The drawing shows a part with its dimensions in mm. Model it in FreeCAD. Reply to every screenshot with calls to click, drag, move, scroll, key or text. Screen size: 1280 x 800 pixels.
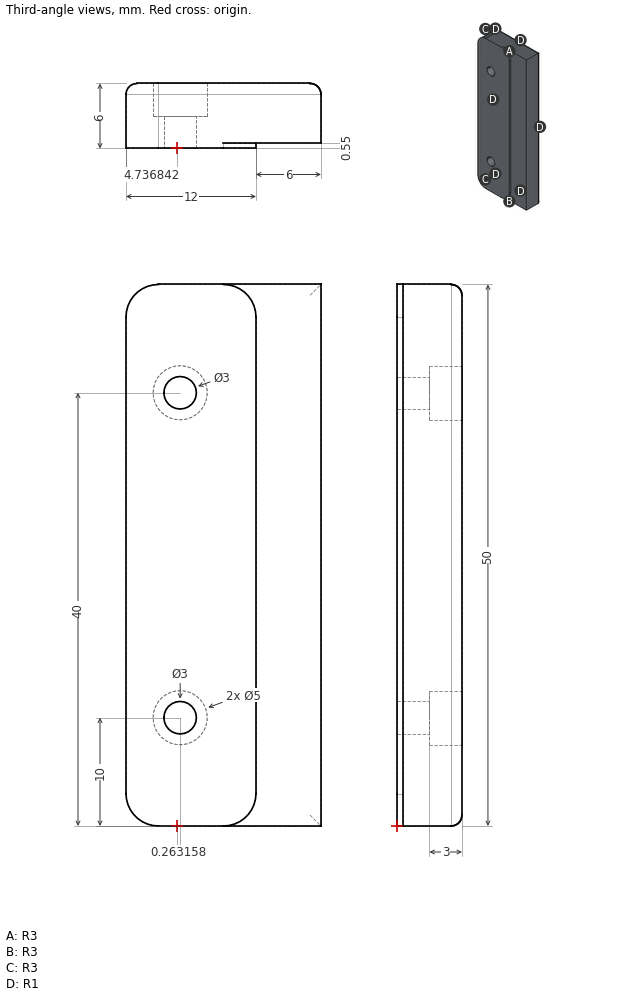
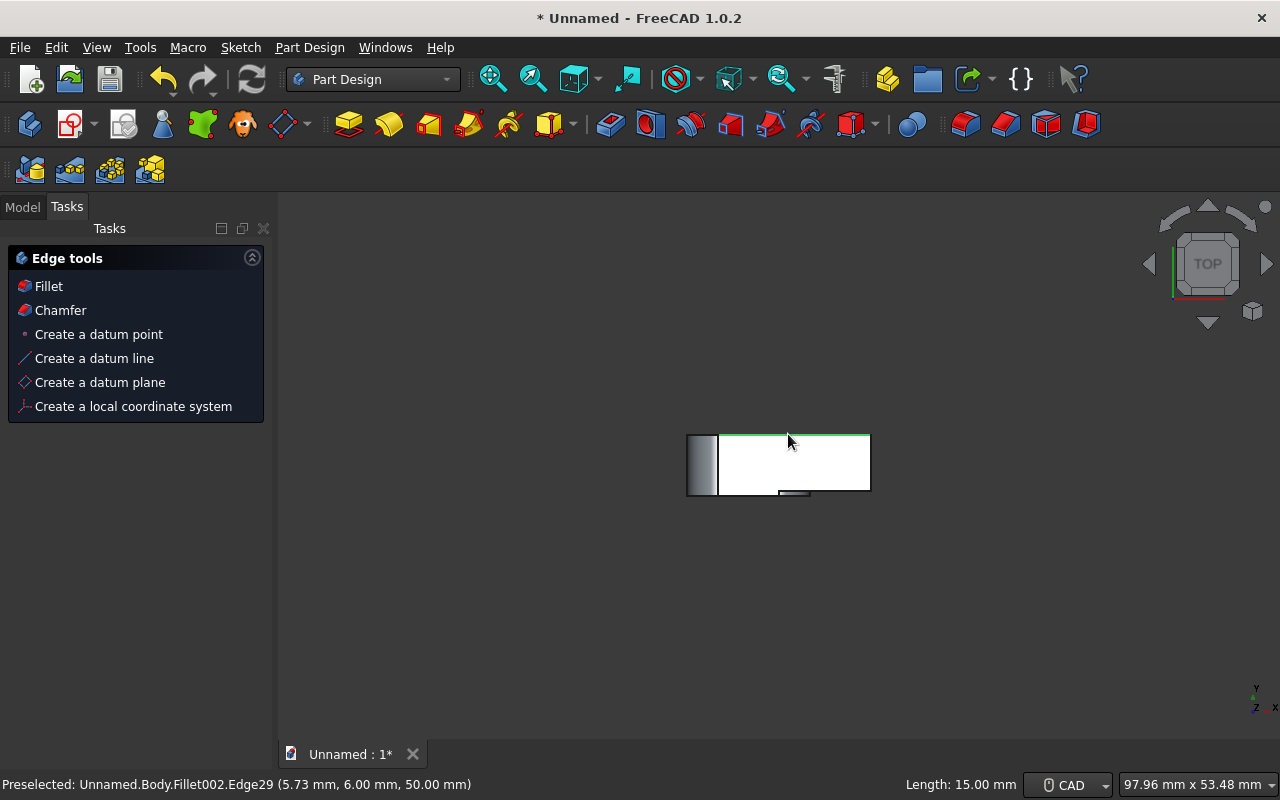
click(696, 434, ctrl)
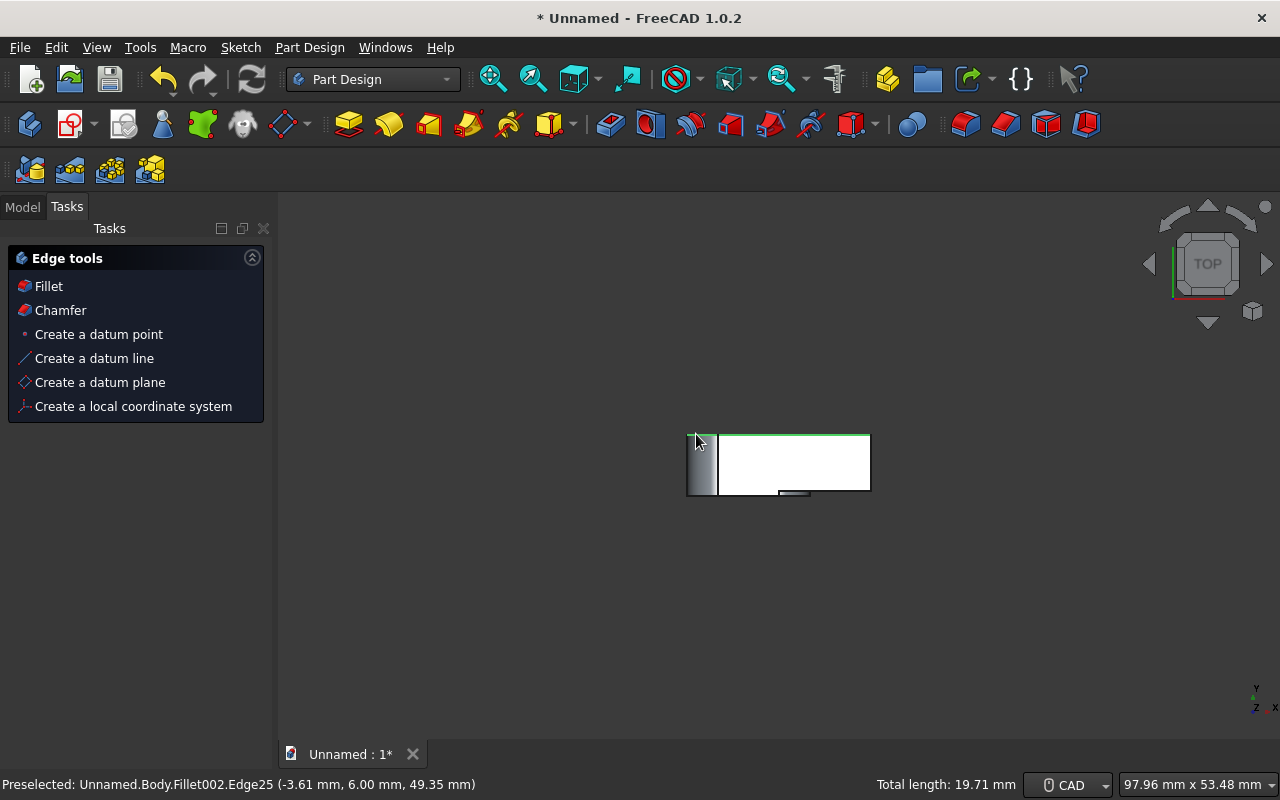
key(0)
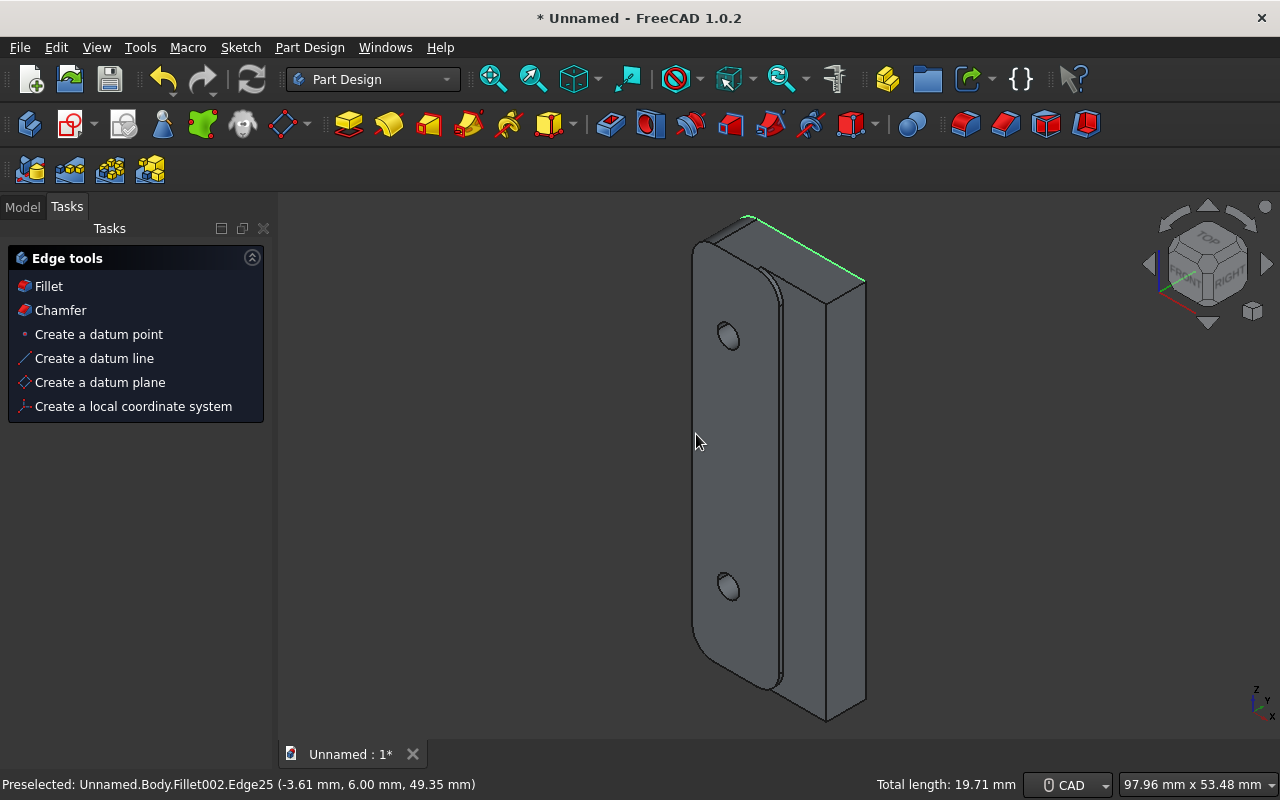
key(1)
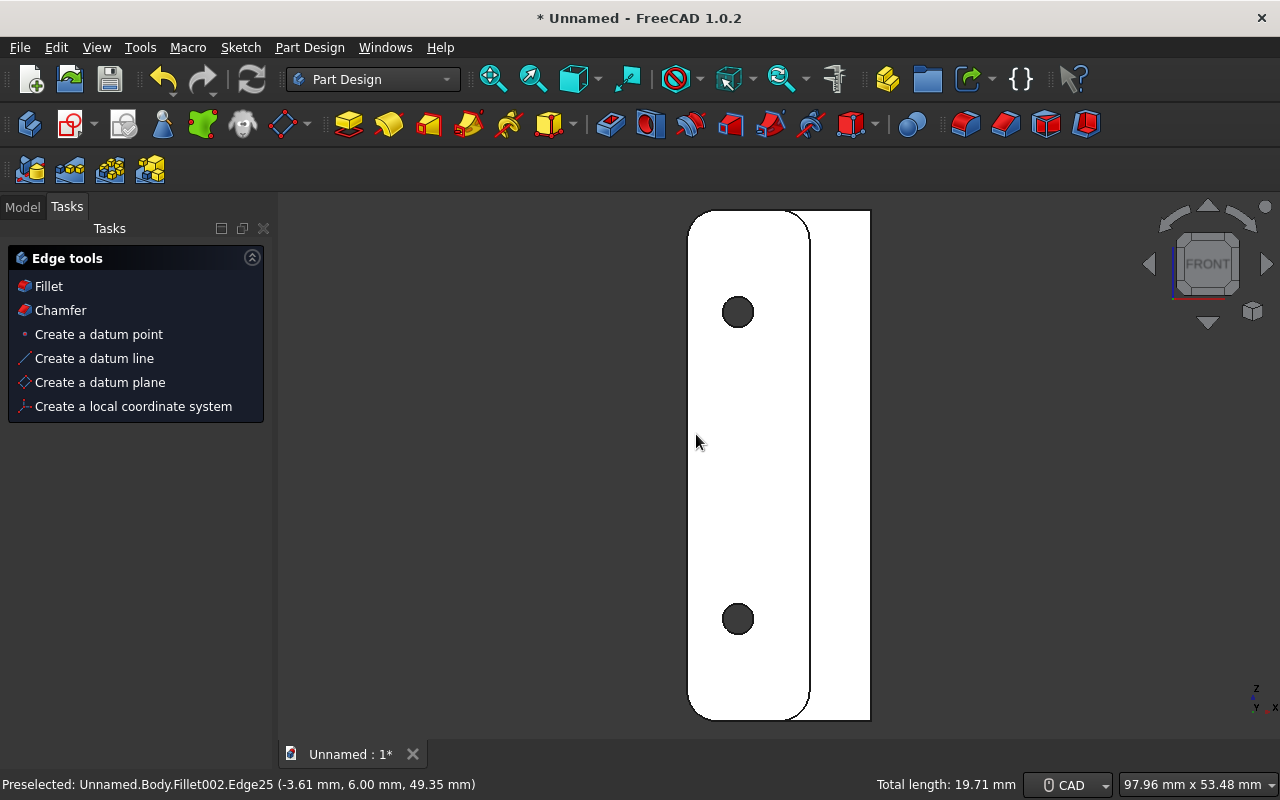
key(3)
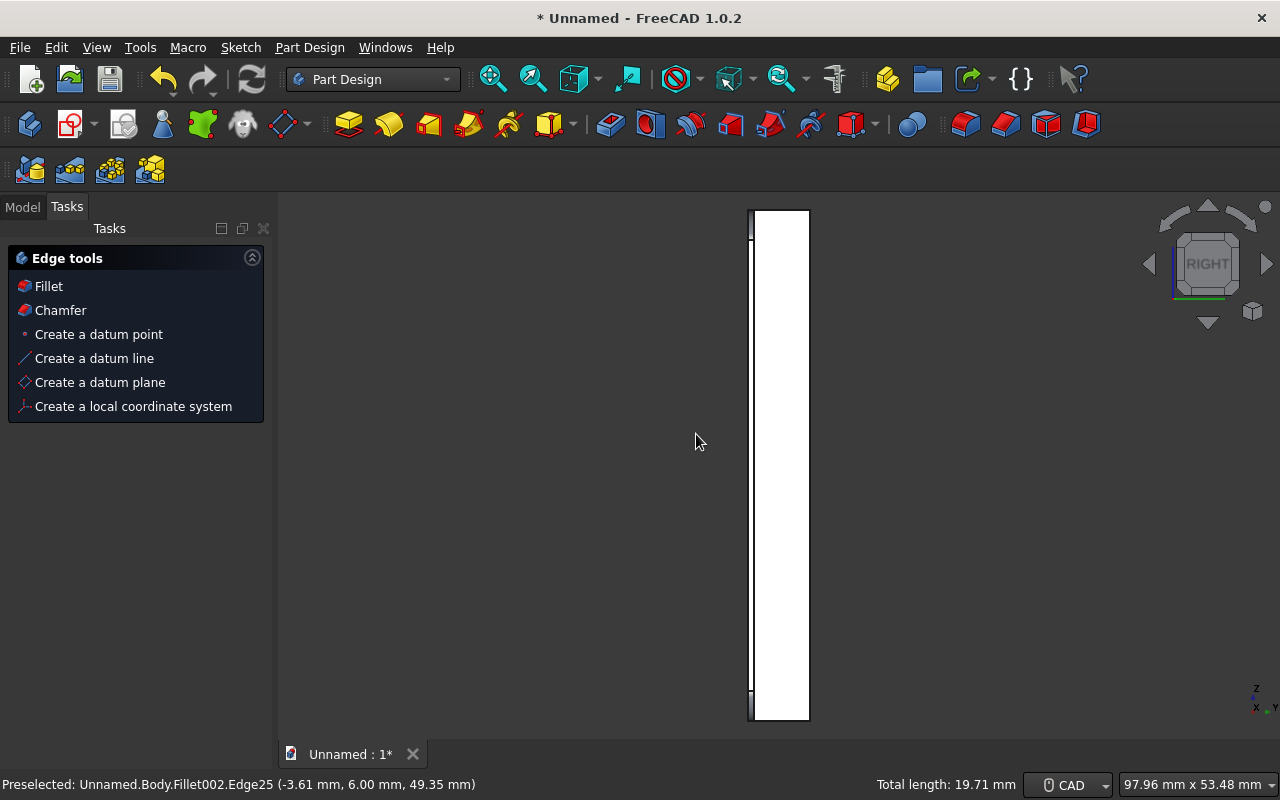
click(810, 464, ctrl)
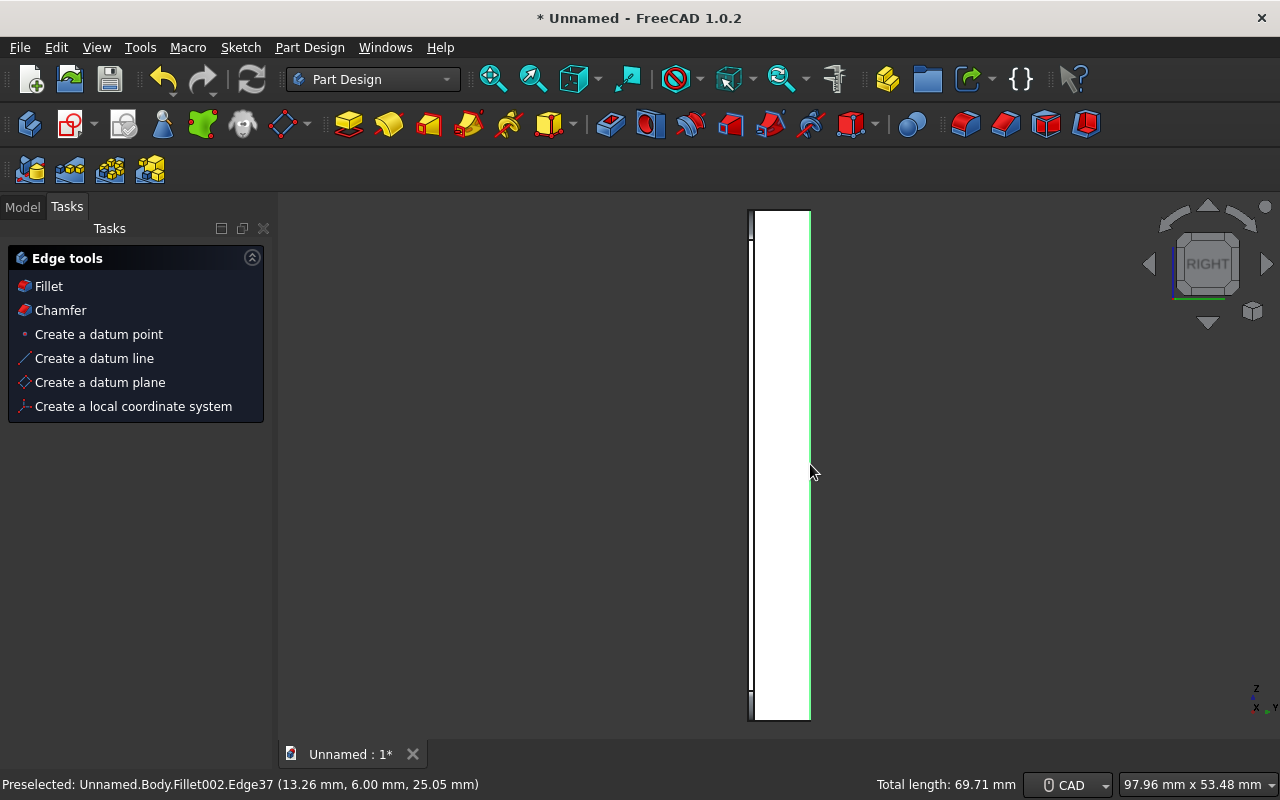
key(5)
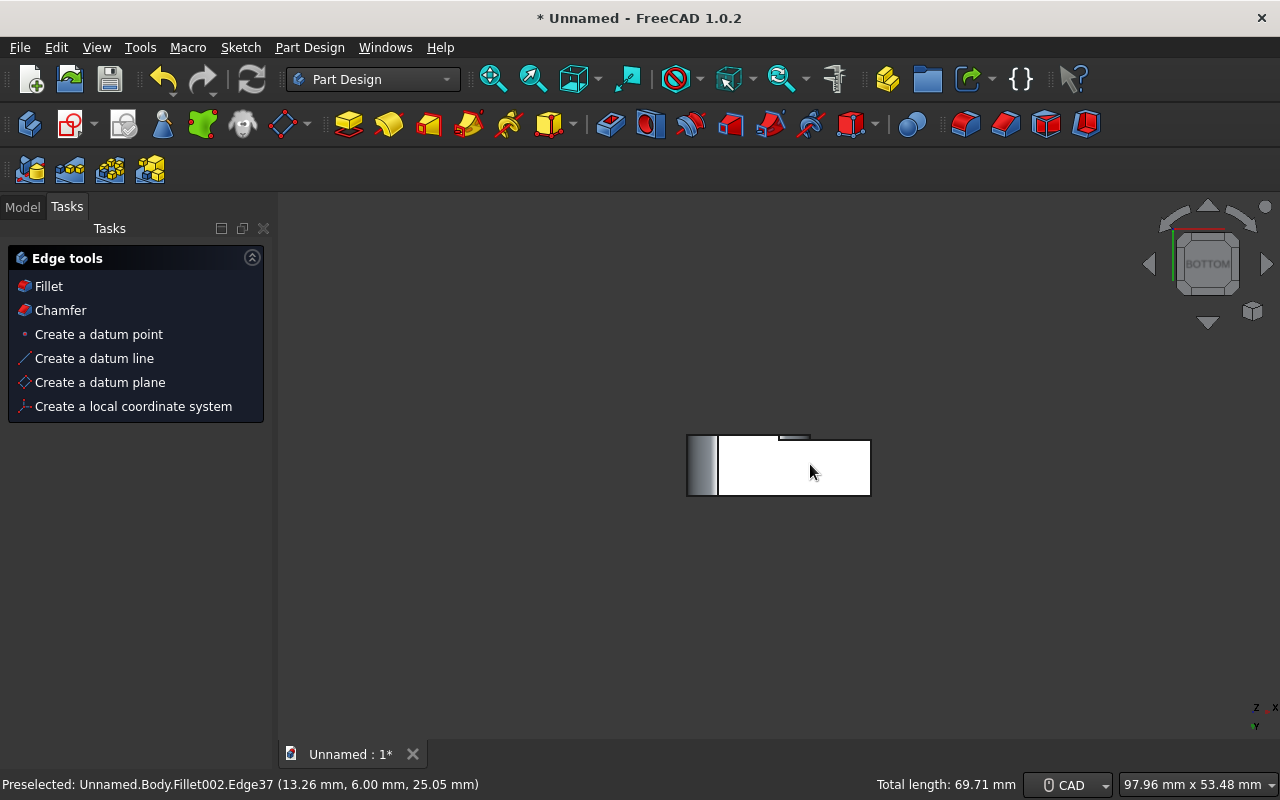
click(494, 80)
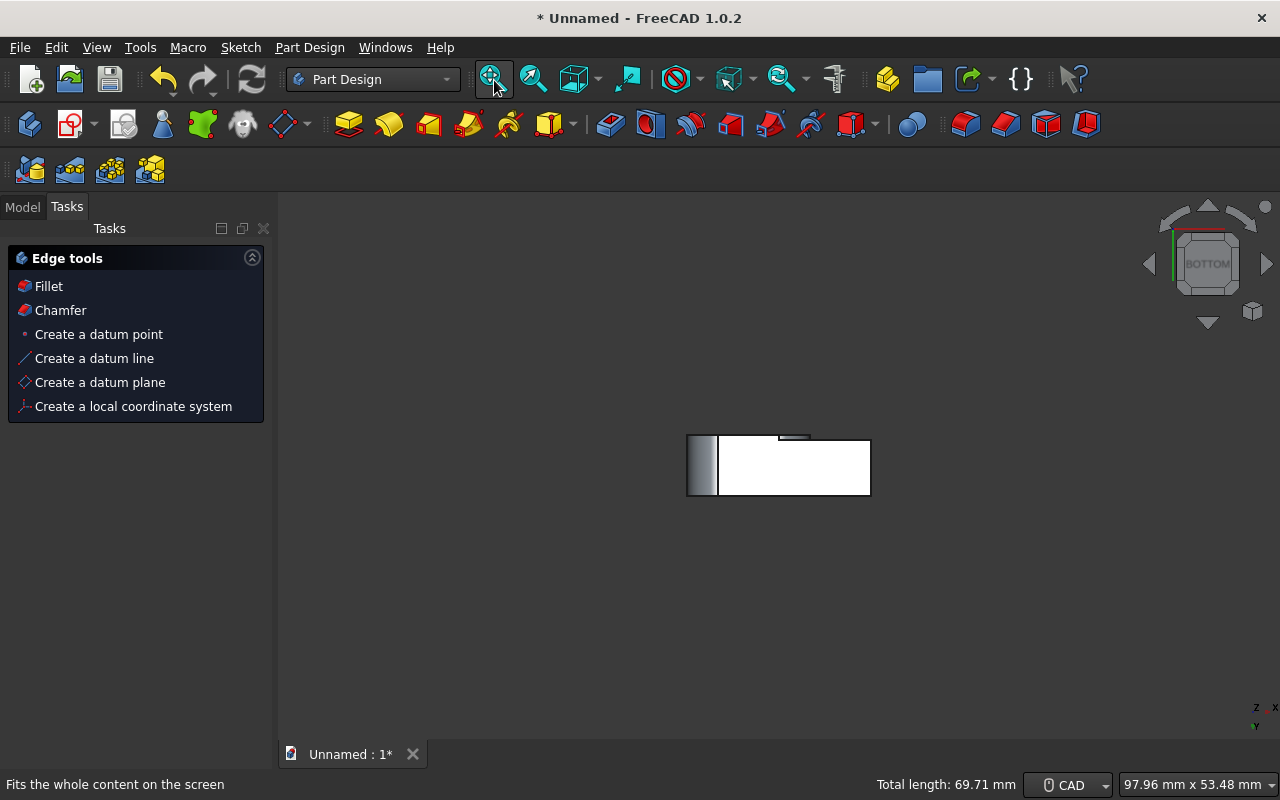
click(696, 495, ctrl)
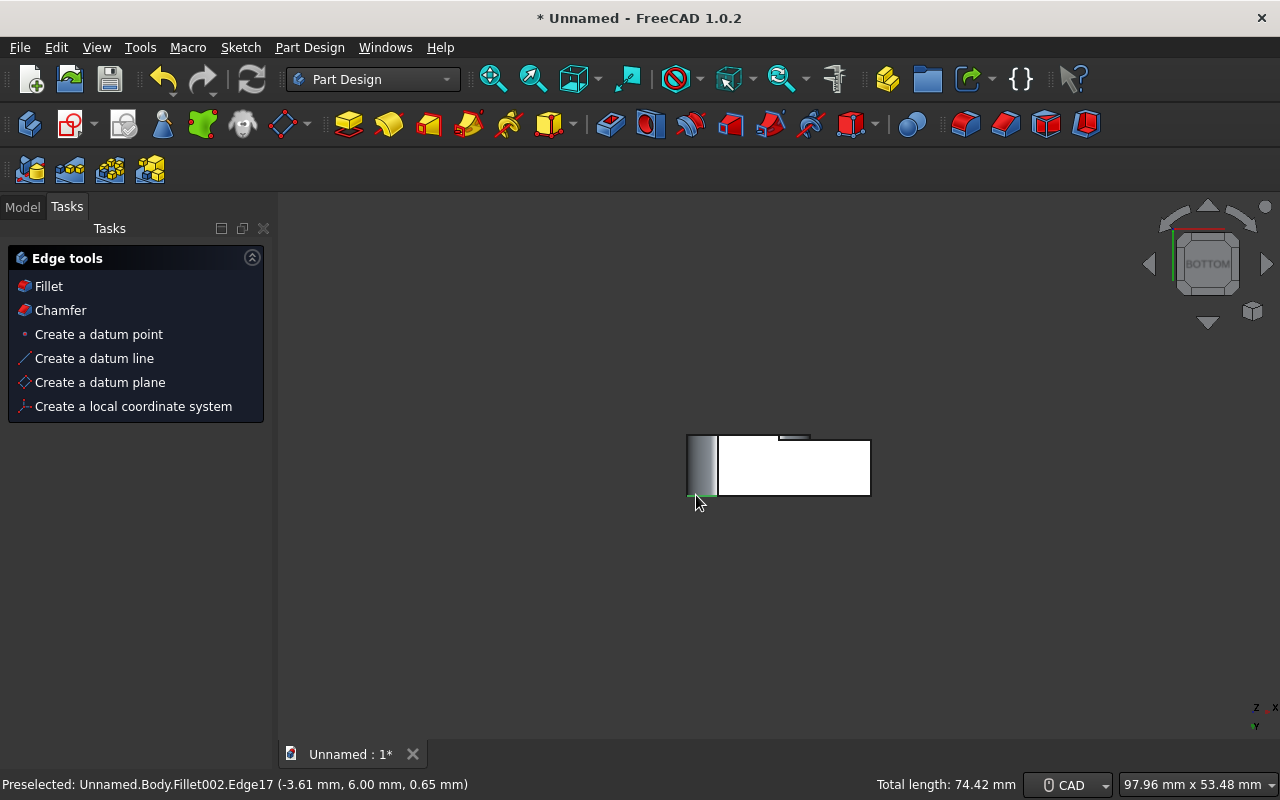
click(794, 495, ctrl)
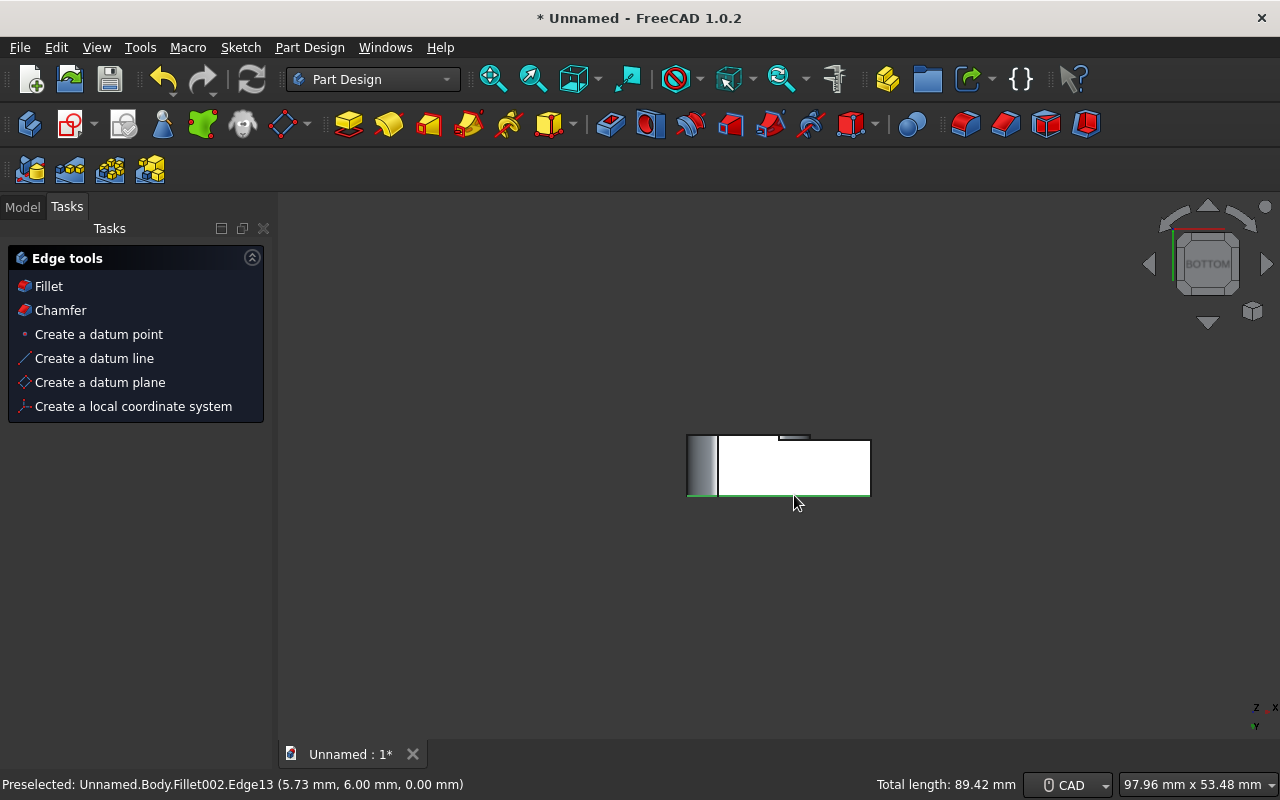
key(4)